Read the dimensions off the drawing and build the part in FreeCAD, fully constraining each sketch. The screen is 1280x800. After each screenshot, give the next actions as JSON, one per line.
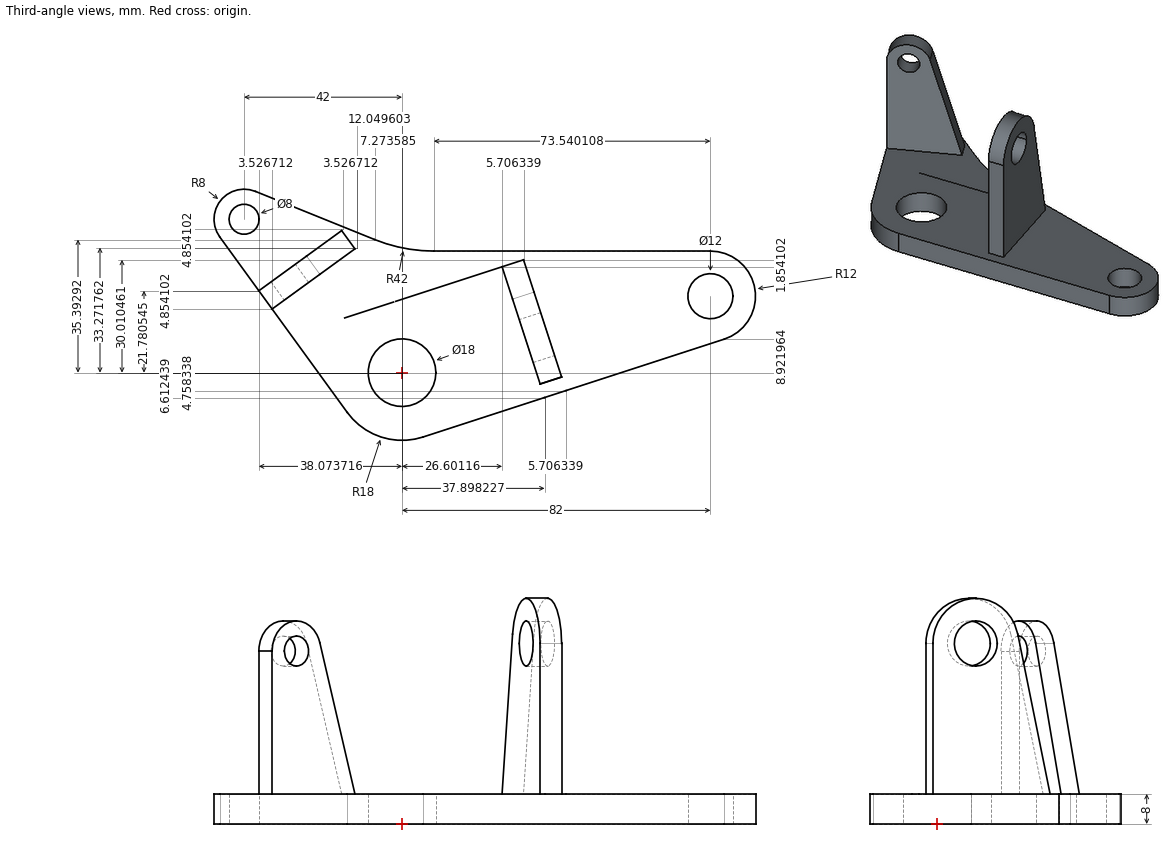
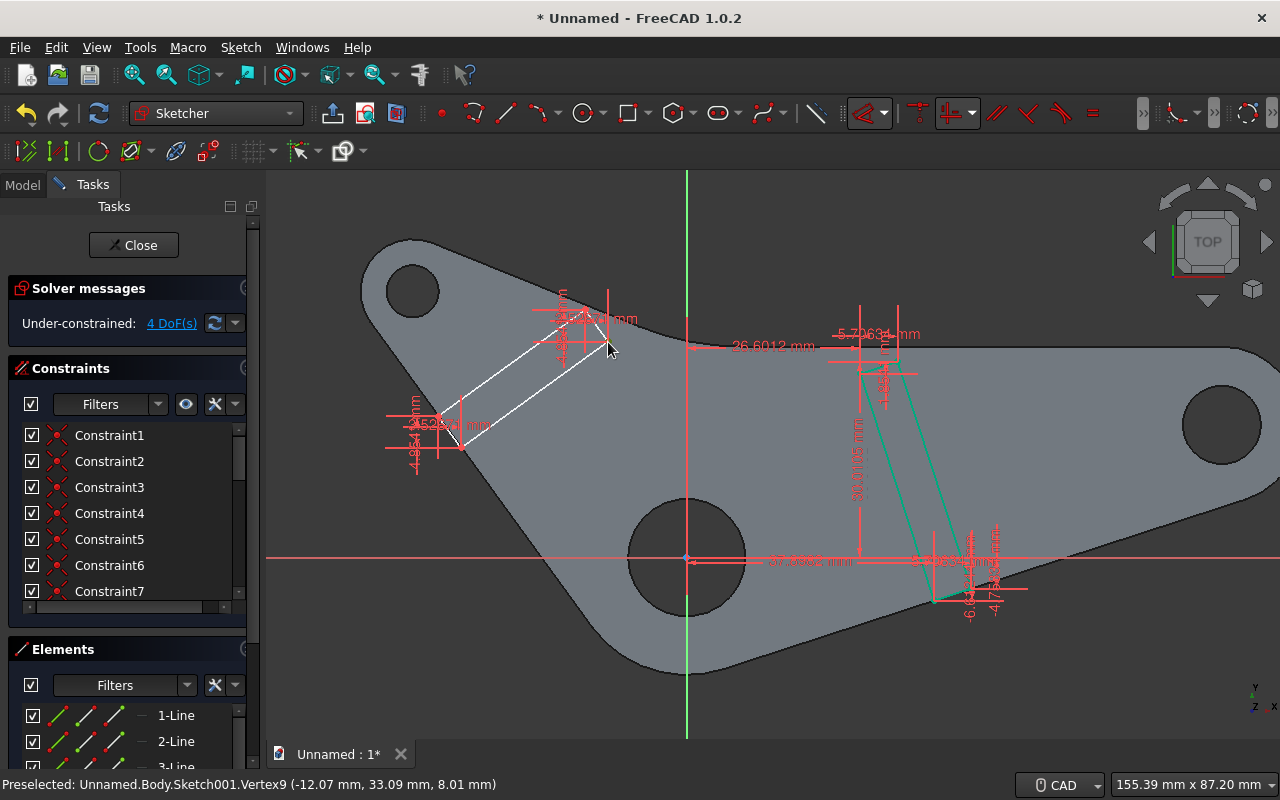
{"action": "key", "text": "l"}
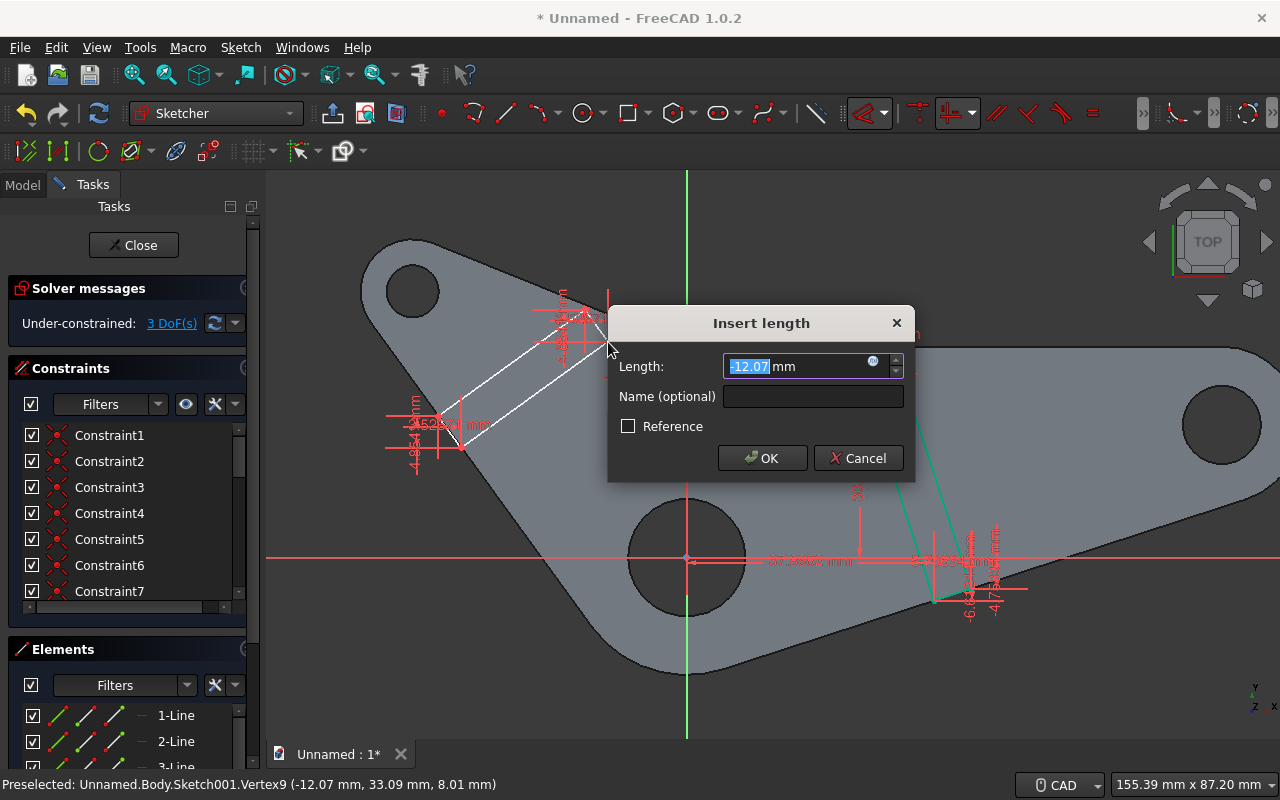
{"action": "type", "text": "-12.049603"}
{"action": "key", "text": "Return"}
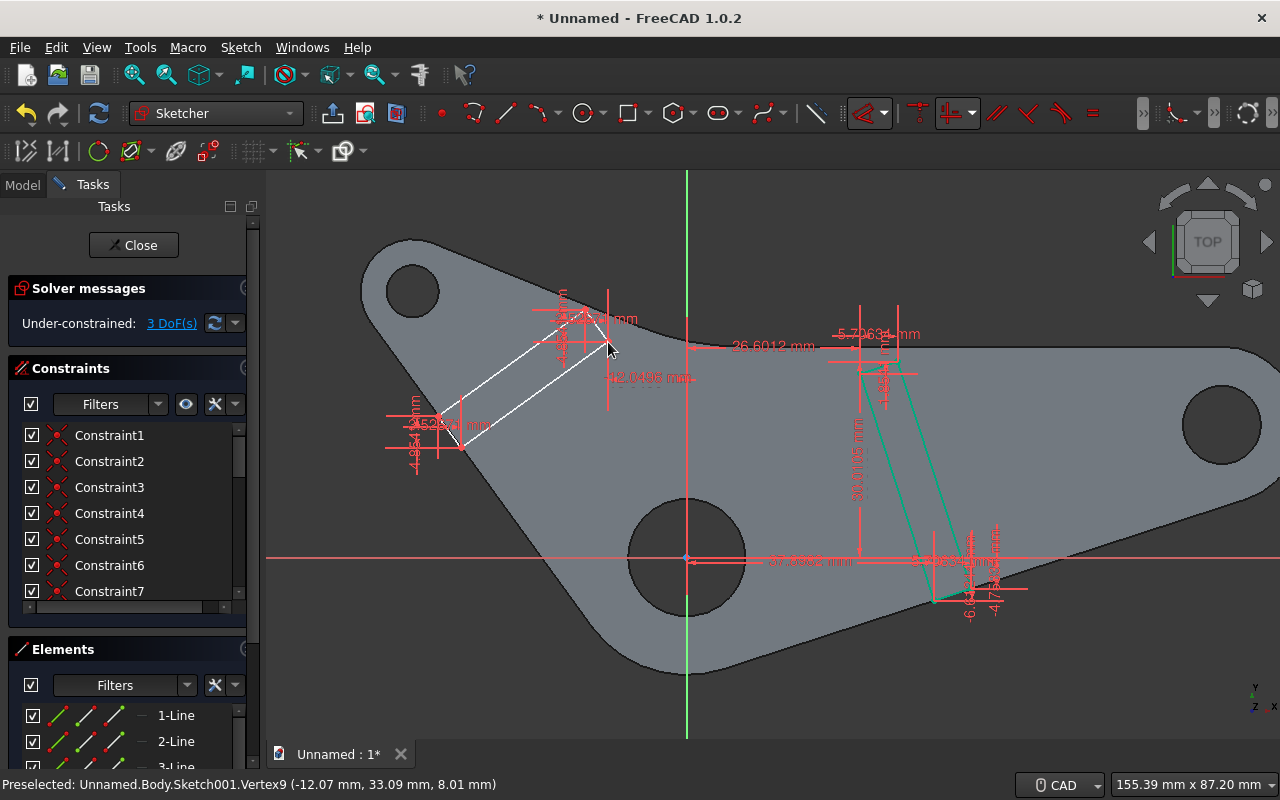
{"action": "left_click", "coordinate": [608, 342]}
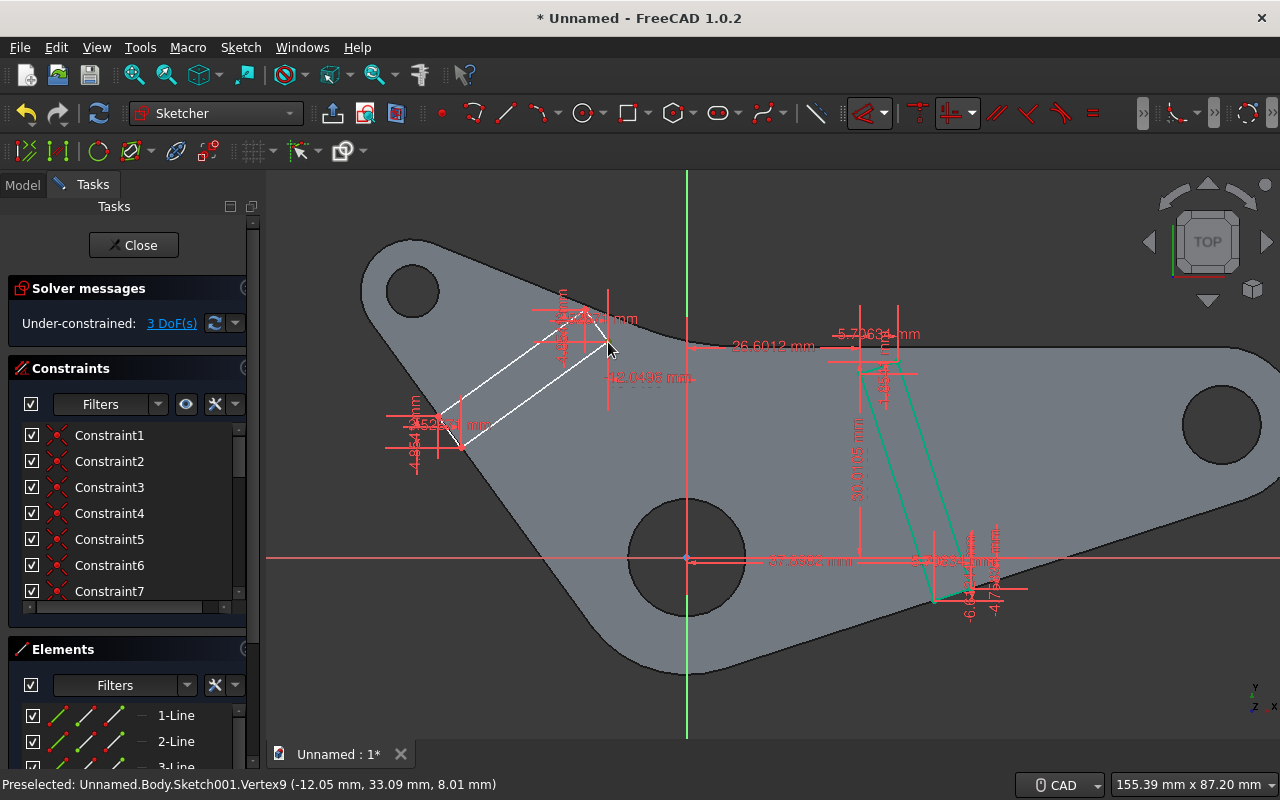
{"action": "left_click", "coordinate": [886, 114]}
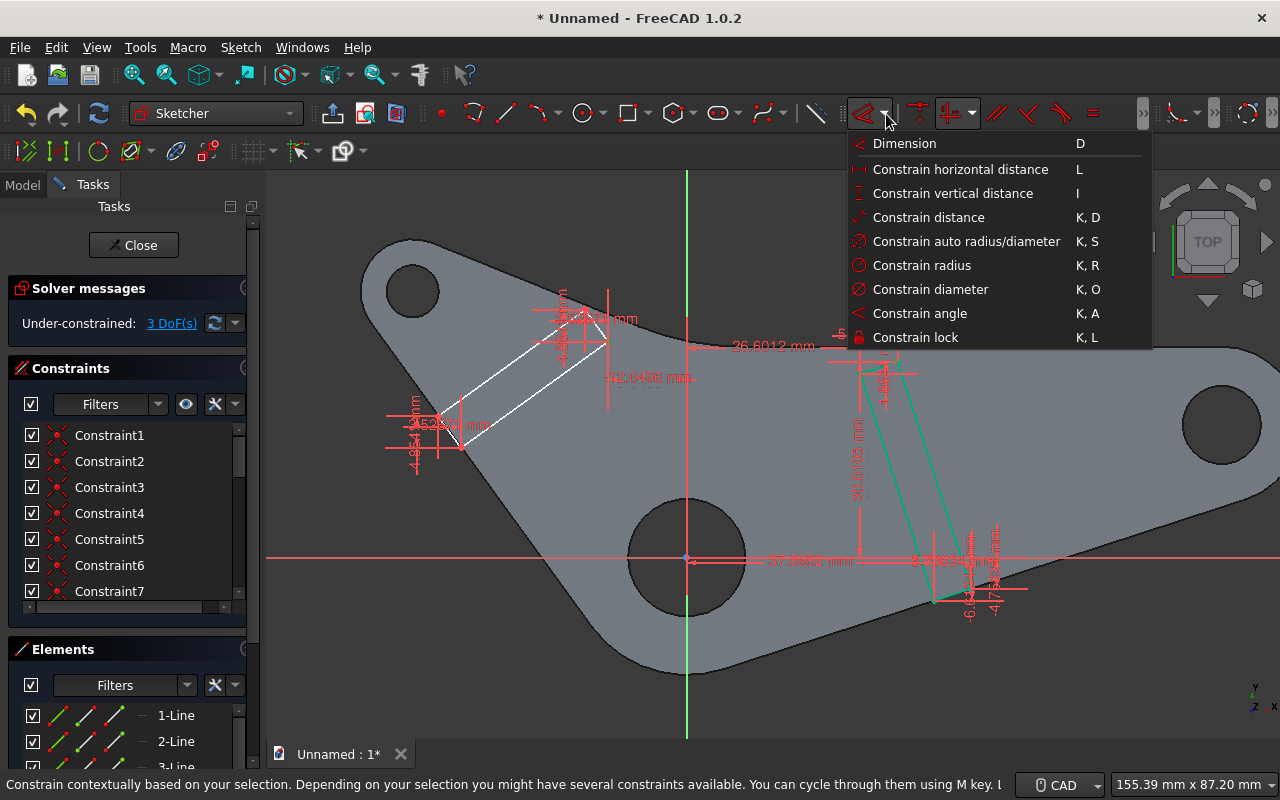
{"action": "left_click", "coordinate": [1000, 193]}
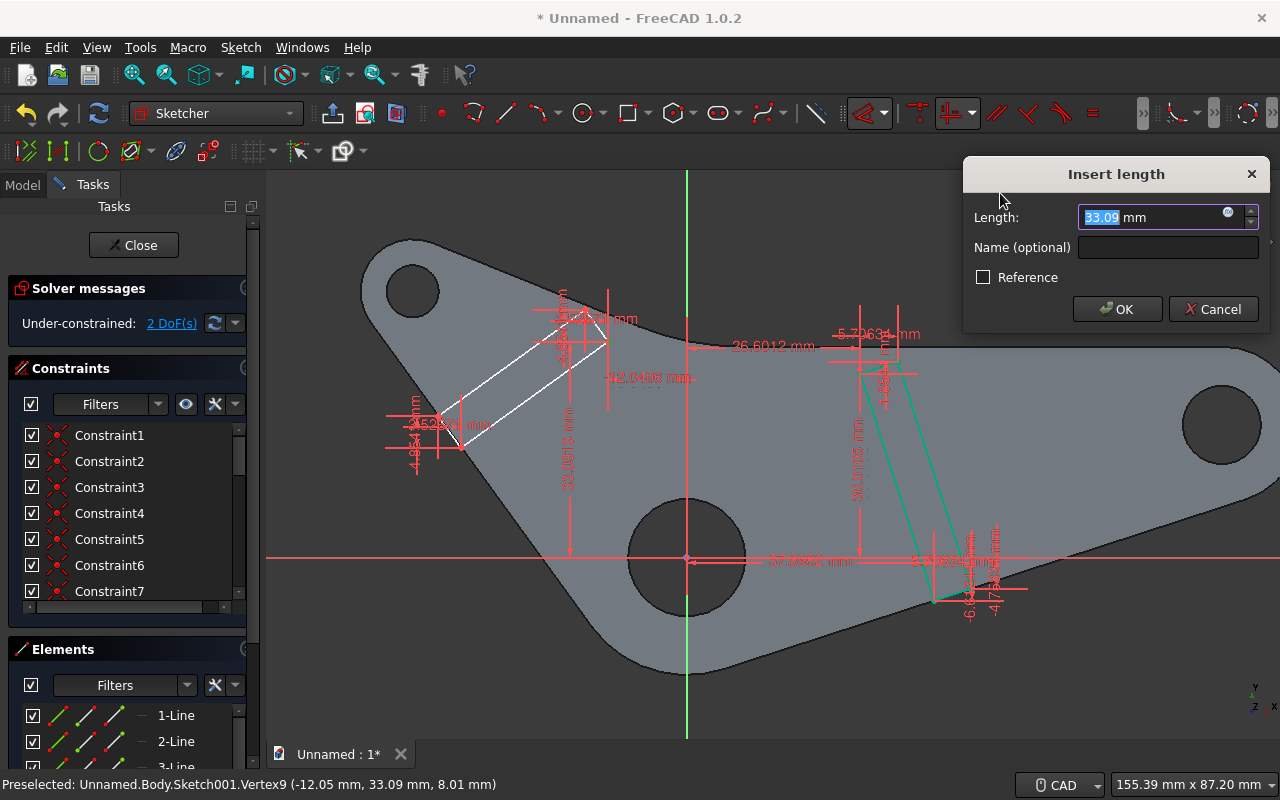
{"action": "type", "text": "33.271762"}
{"action": "key", "text": "Return"}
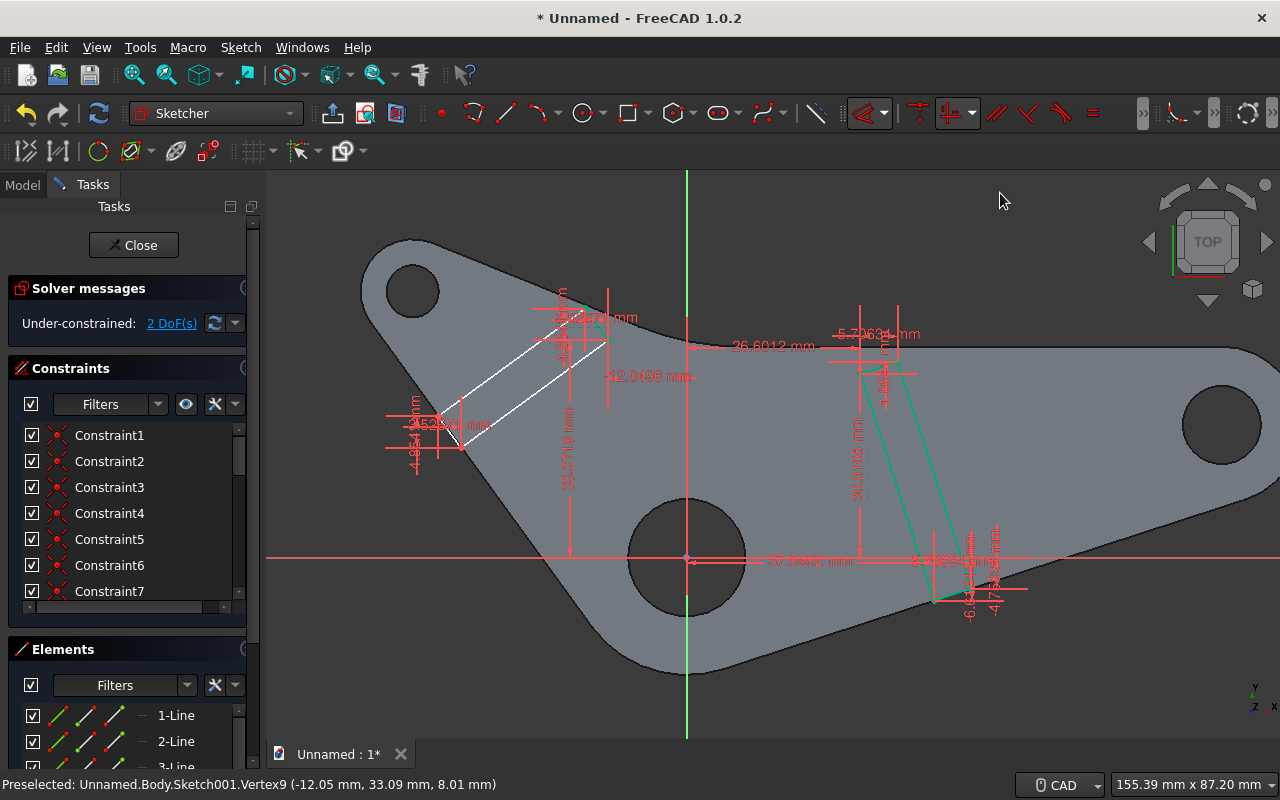
{"action": "left_click", "coordinate": [438, 416]}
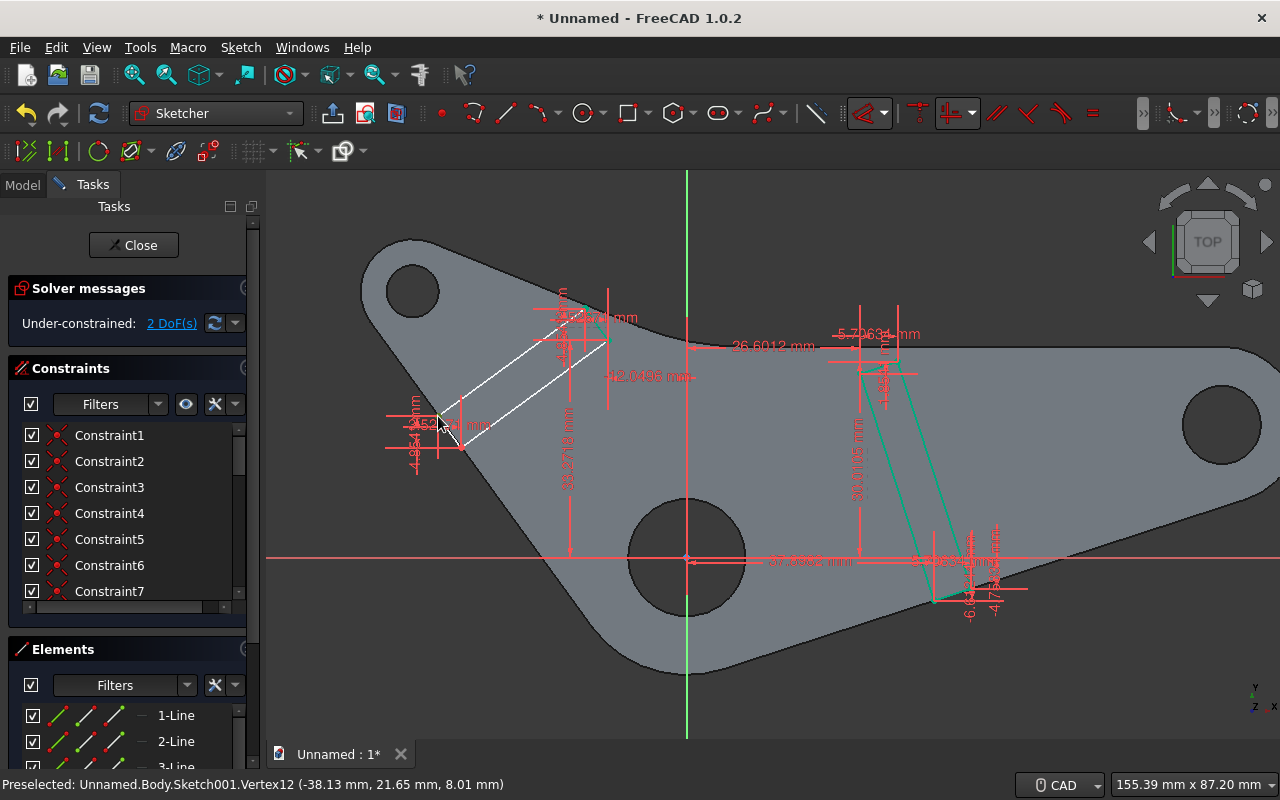
{"action": "left_click", "coordinate": [886, 114]}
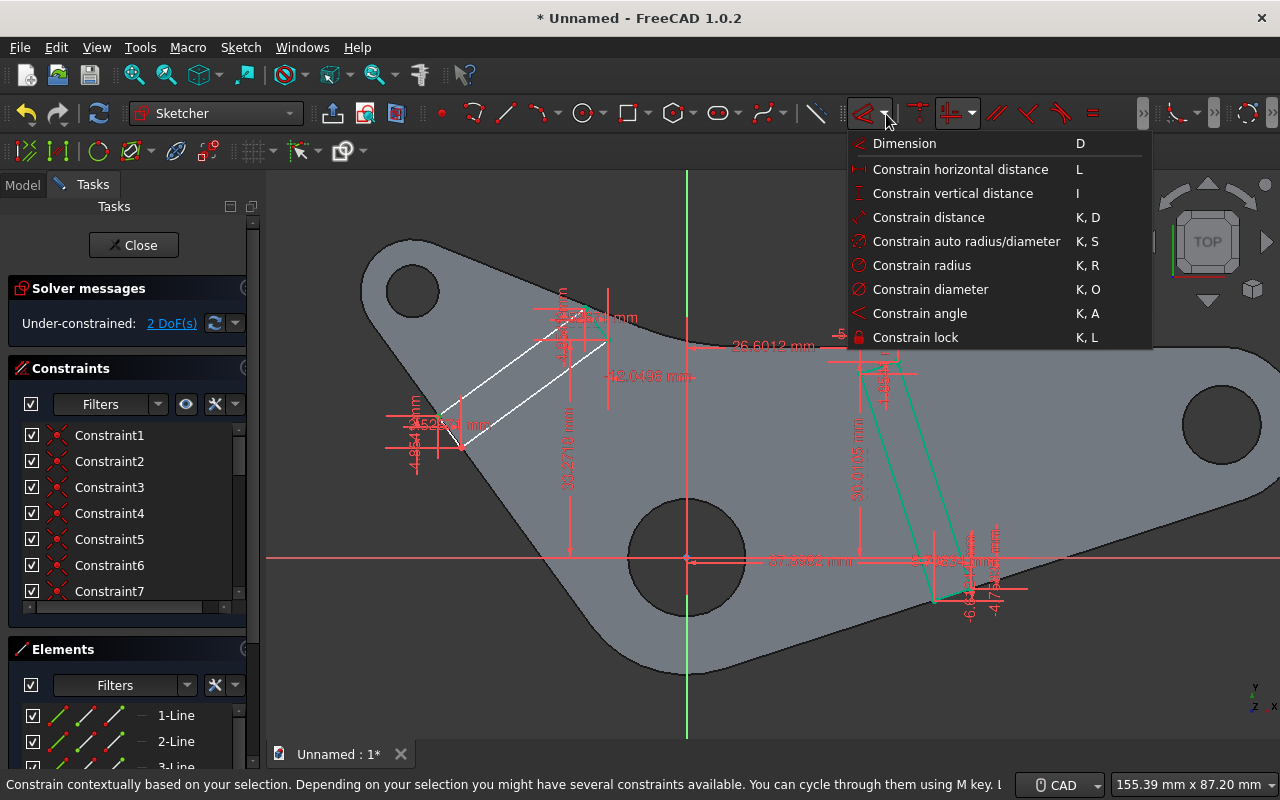
{"action": "left_click", "coordinate": [1000, 169]}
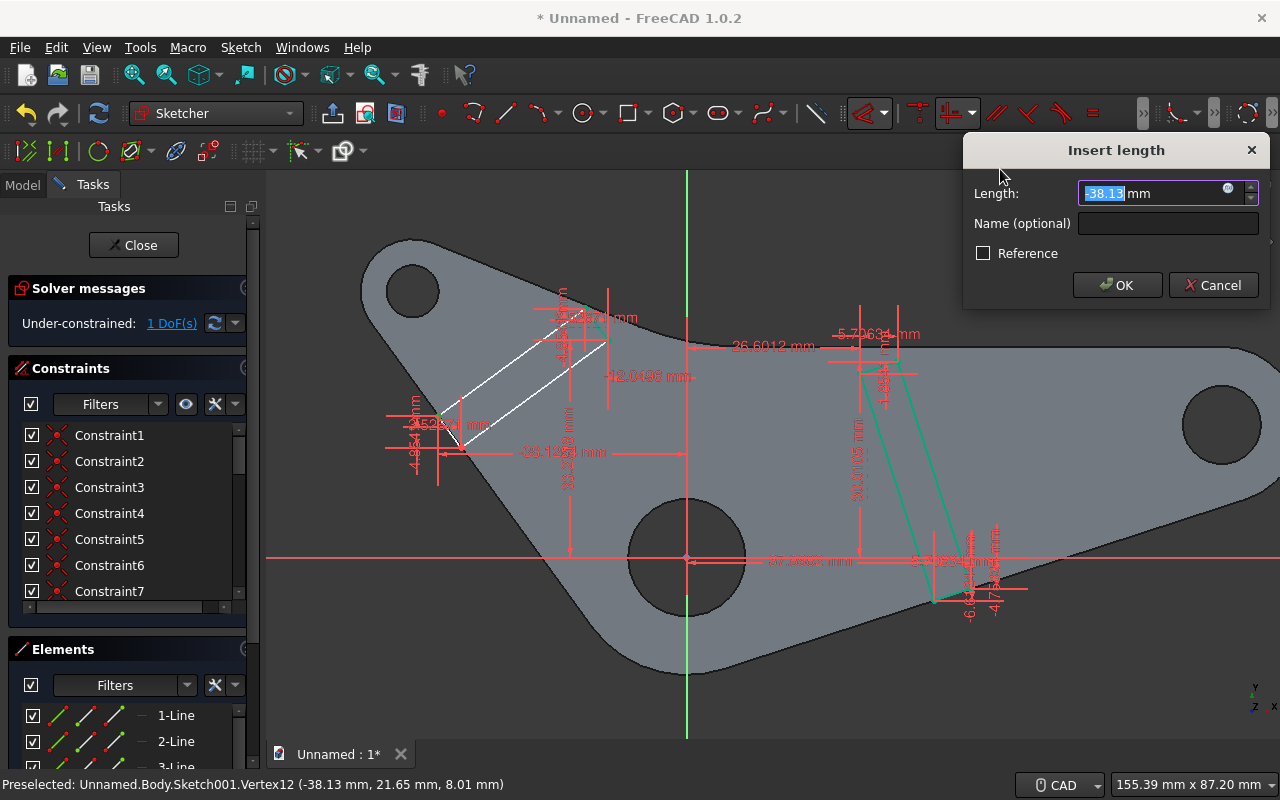
{"action": "type", "text": "-38.073716"}
{"action": "key", "text": "Return"}